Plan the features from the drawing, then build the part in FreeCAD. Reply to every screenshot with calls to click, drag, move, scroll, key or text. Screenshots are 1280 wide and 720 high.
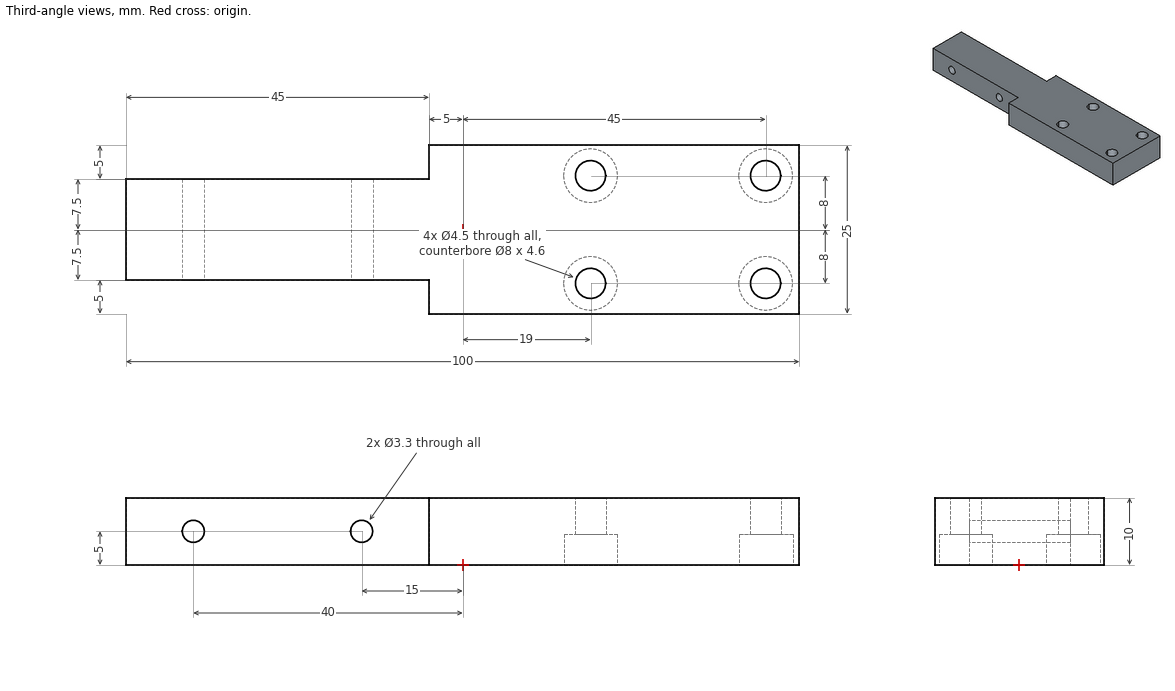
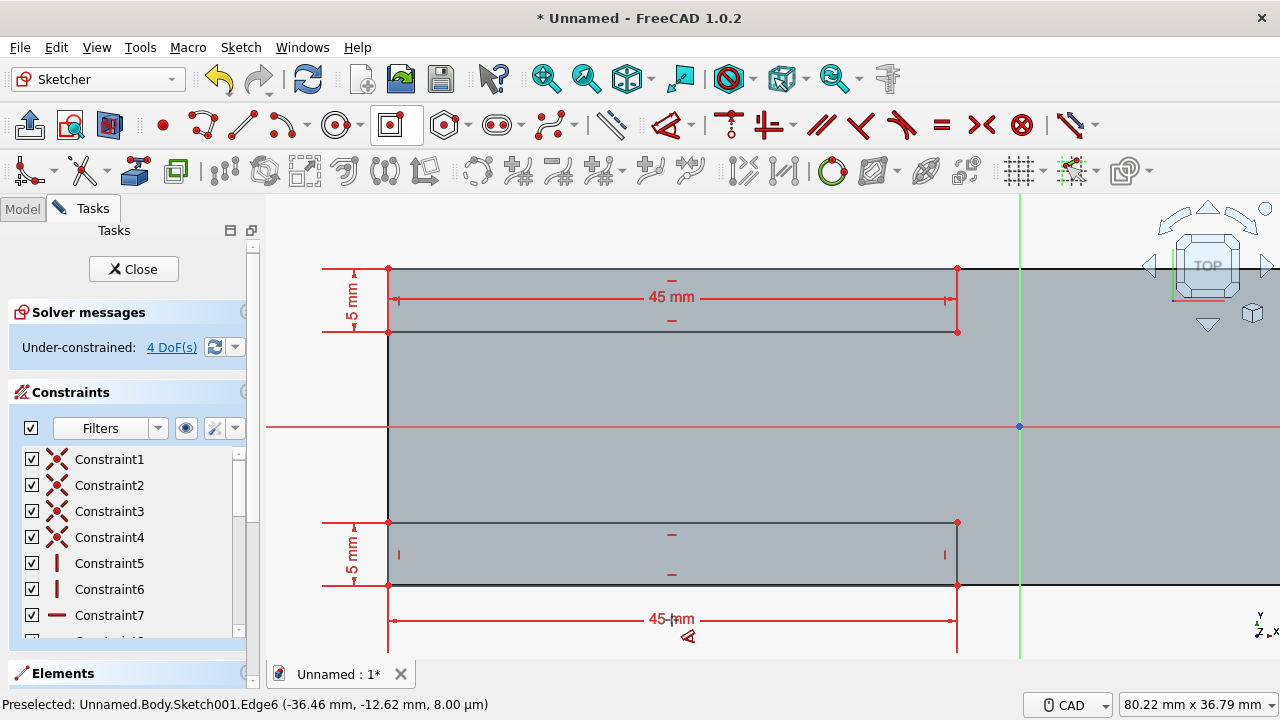
click(957, 332)
click(988, 298)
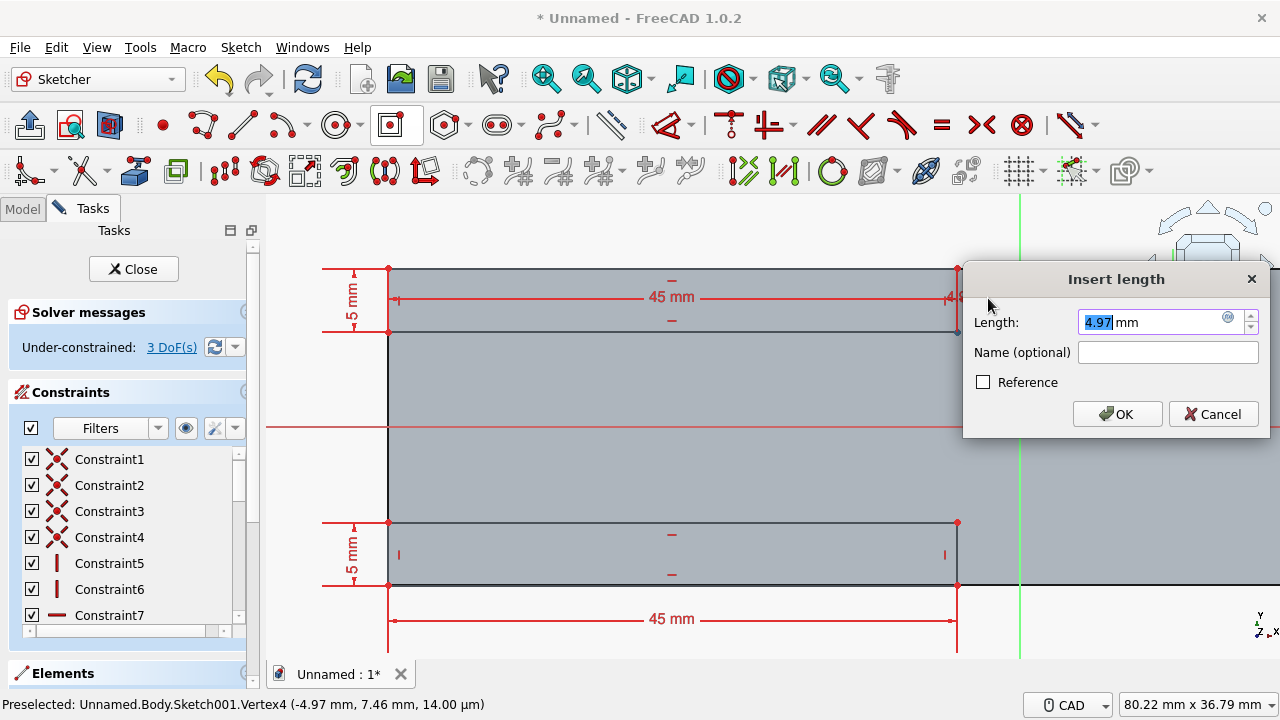
text(5)
key(Return)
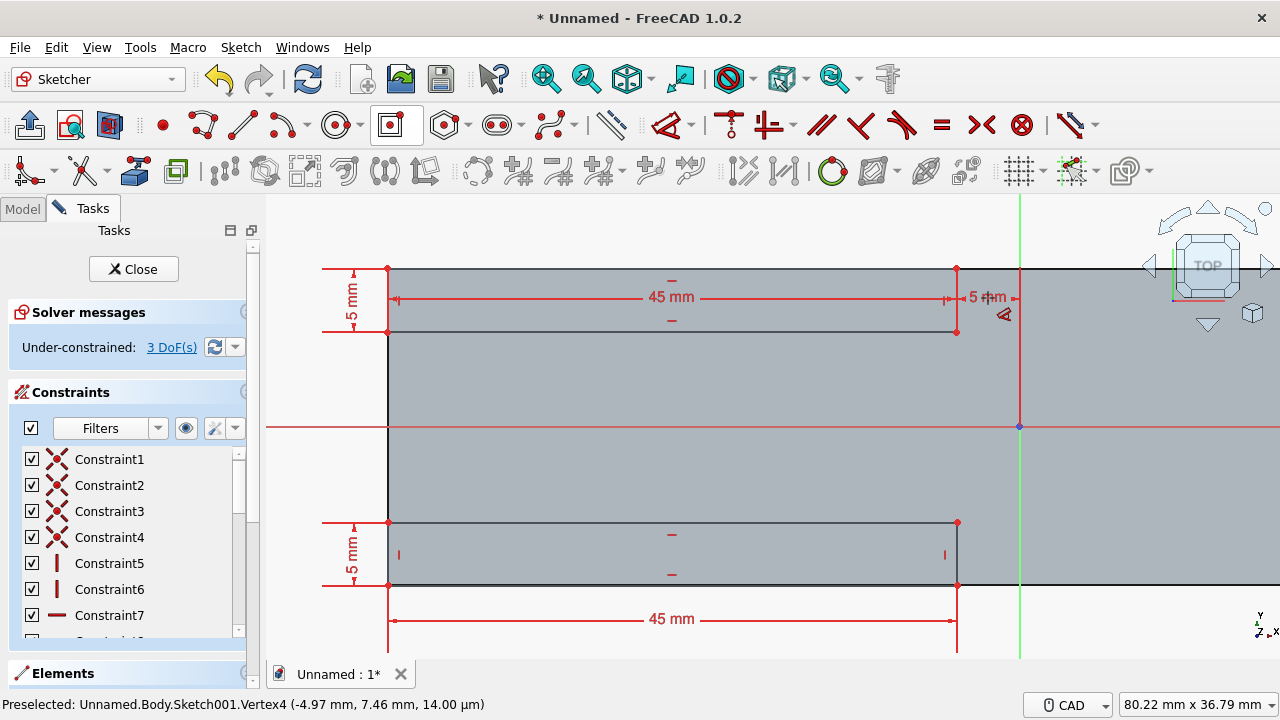
click(957, 586)
click(988, 620)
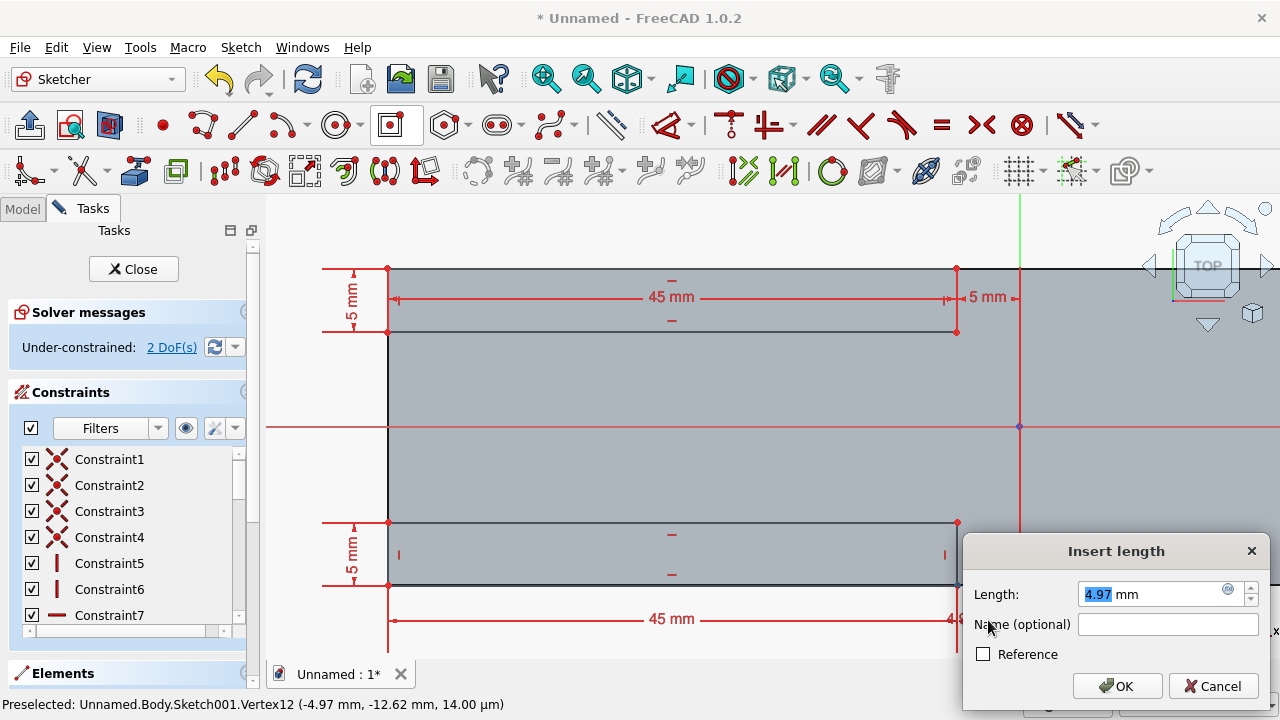
text(5)
key(Return)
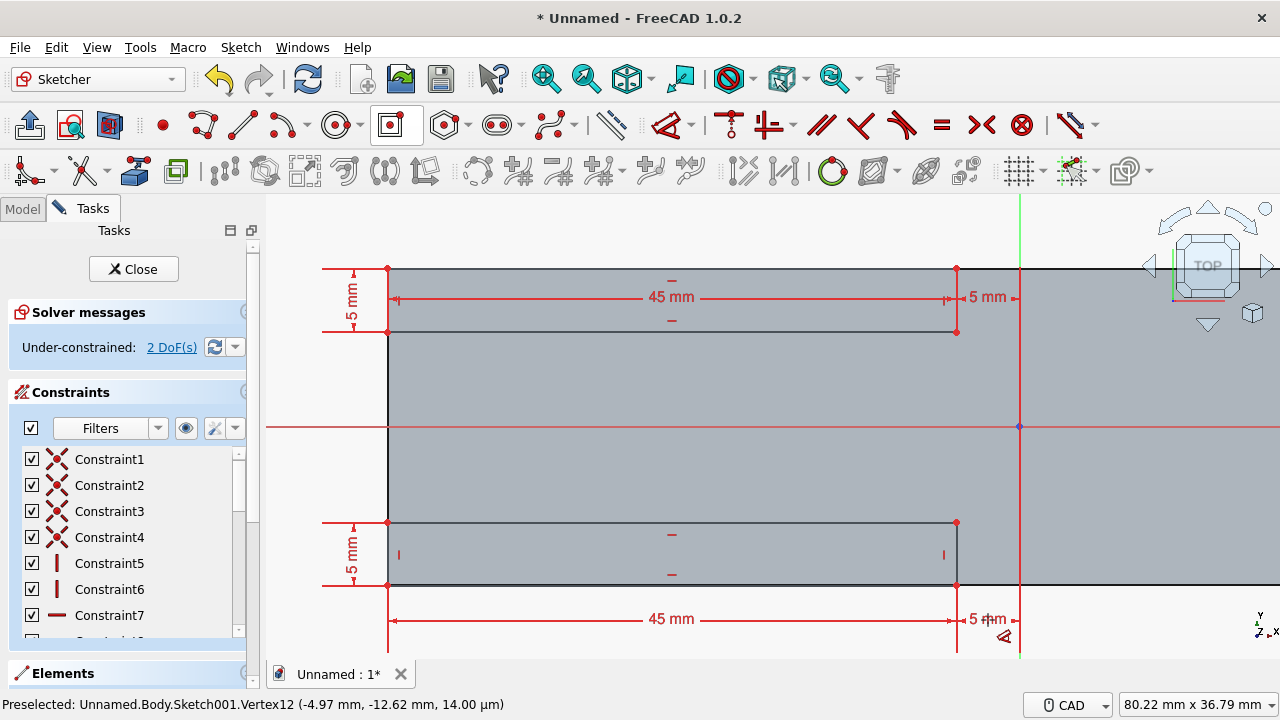
click(388, 332)
click(1054, 379)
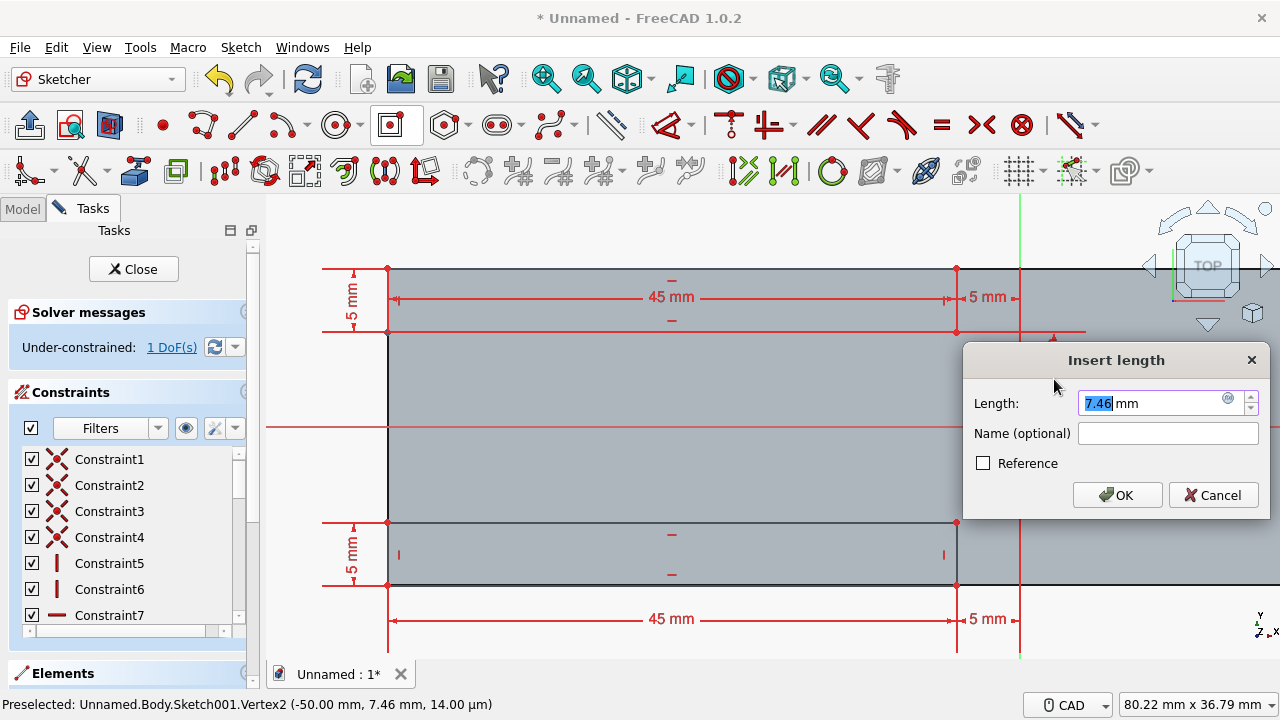
text(7.5)
key(Return)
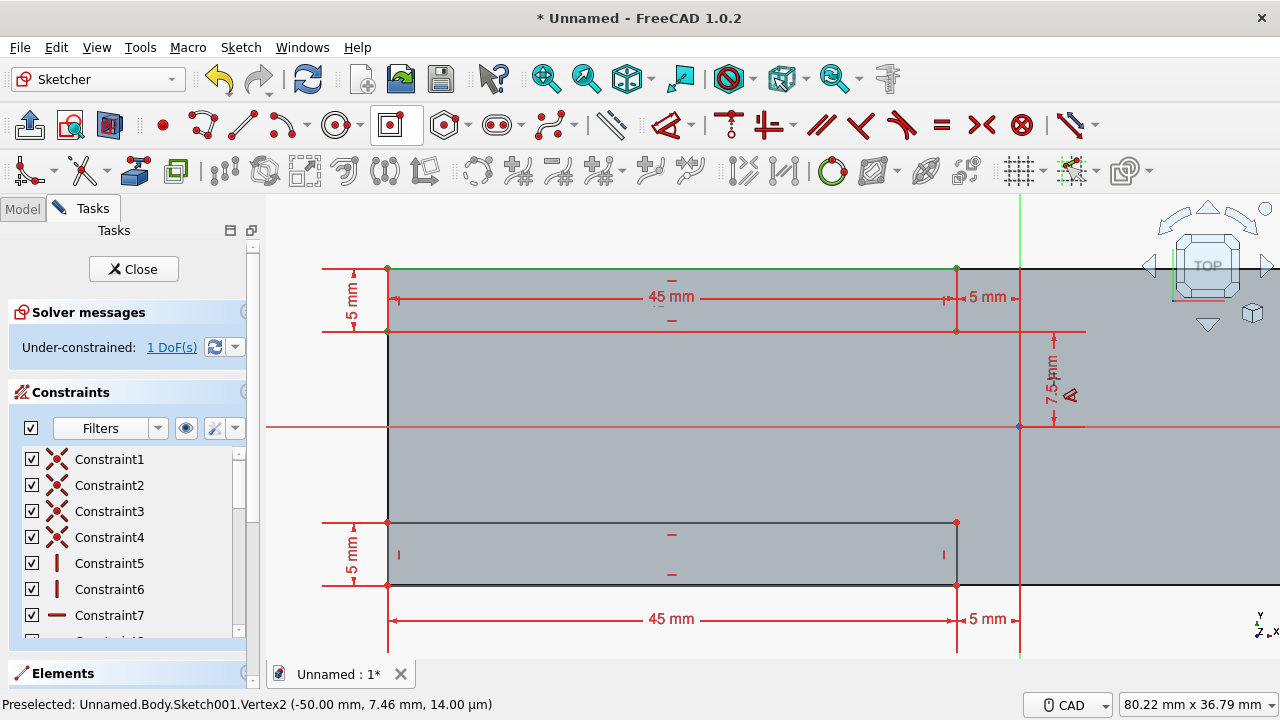
click(388, 523)
click(1054, 475)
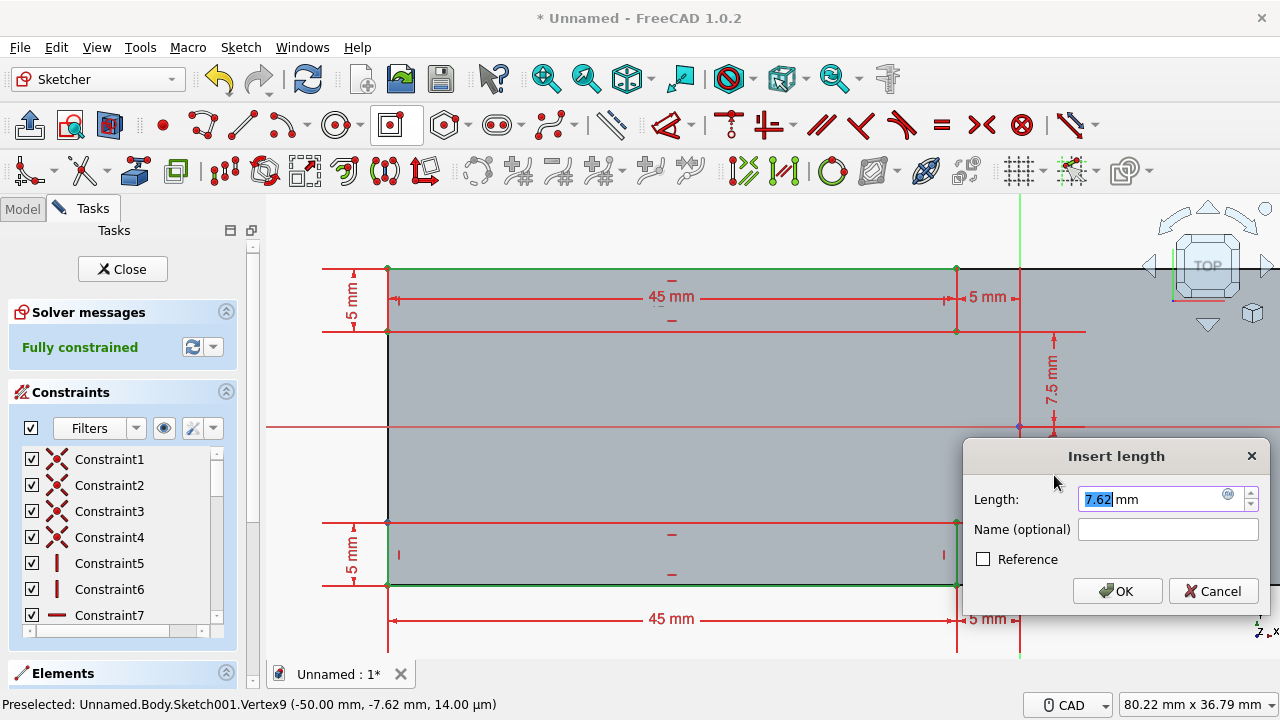
text(7.5)
key(Return)
key(Escape)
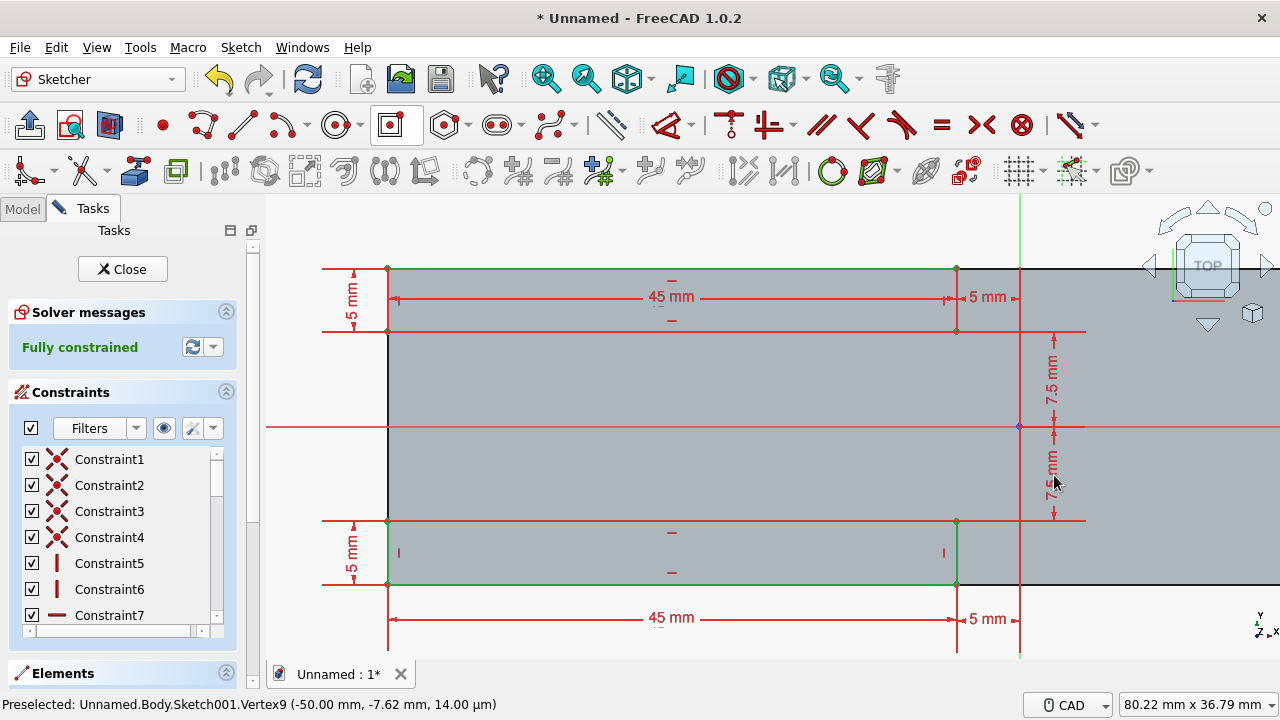
click(123, 269)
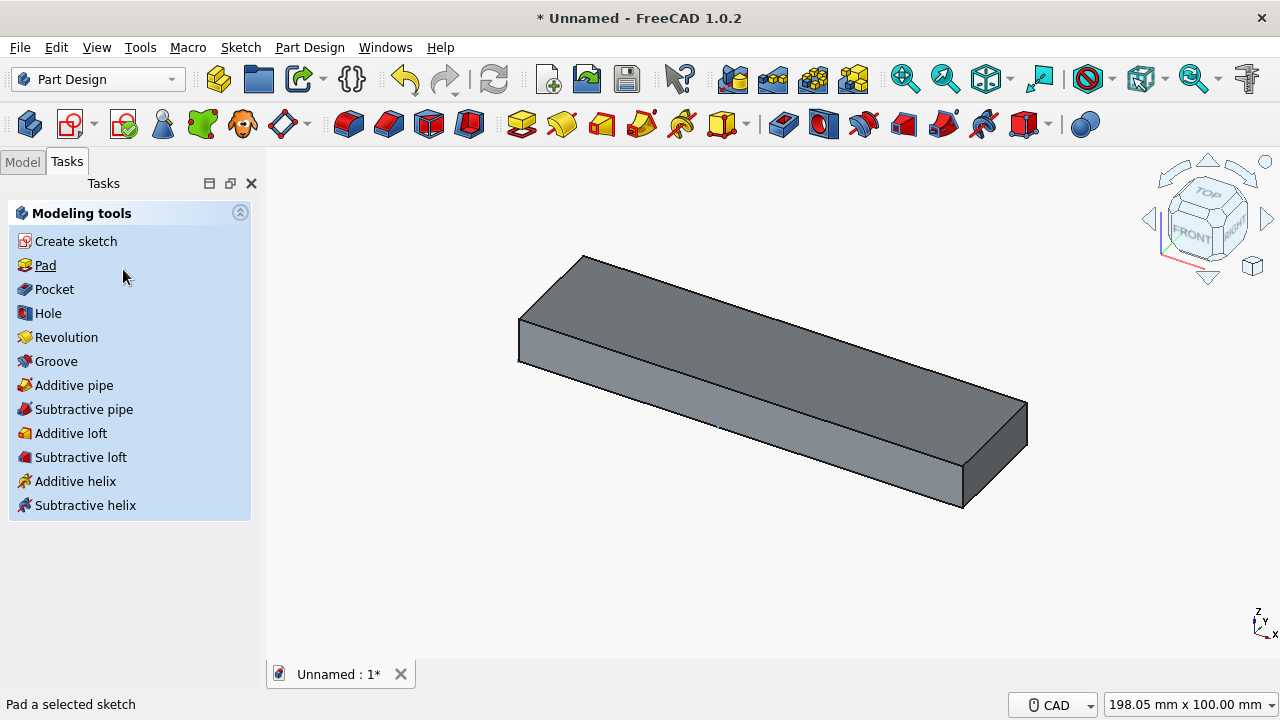
click(784, 124)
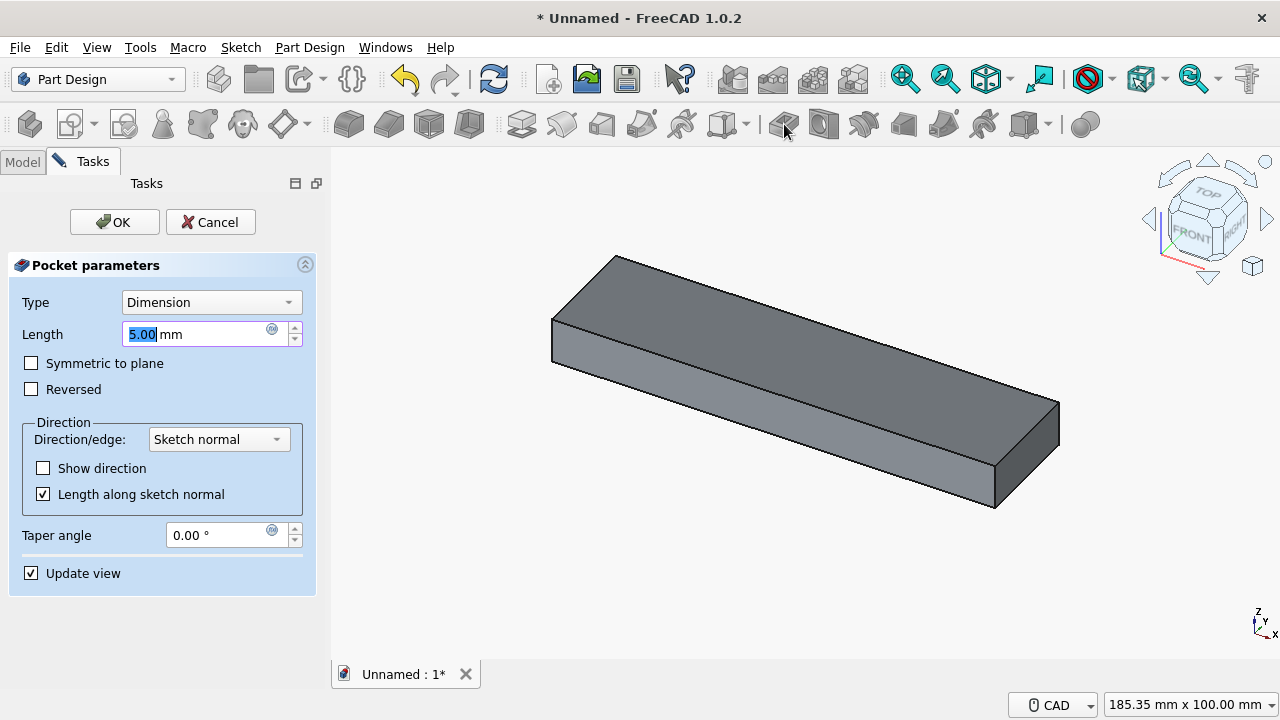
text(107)
key(Tab)